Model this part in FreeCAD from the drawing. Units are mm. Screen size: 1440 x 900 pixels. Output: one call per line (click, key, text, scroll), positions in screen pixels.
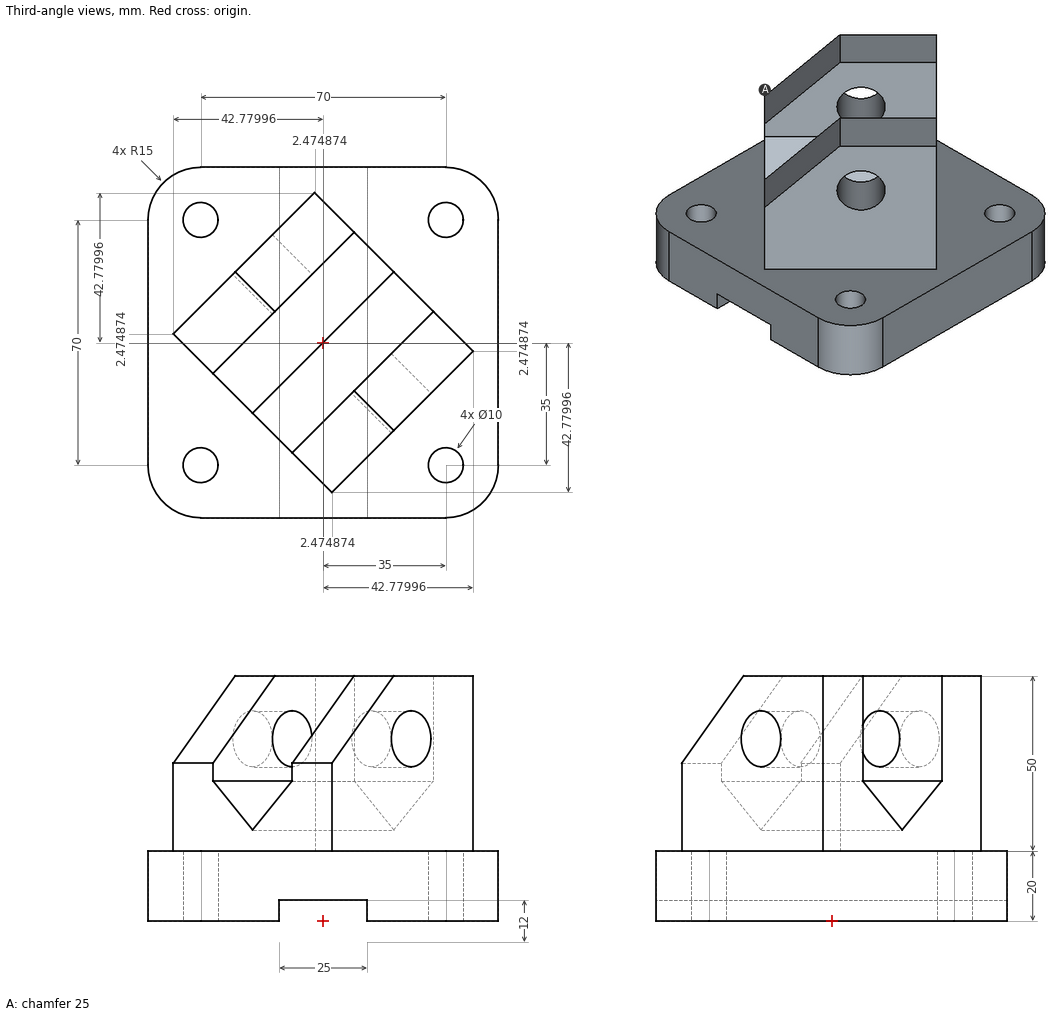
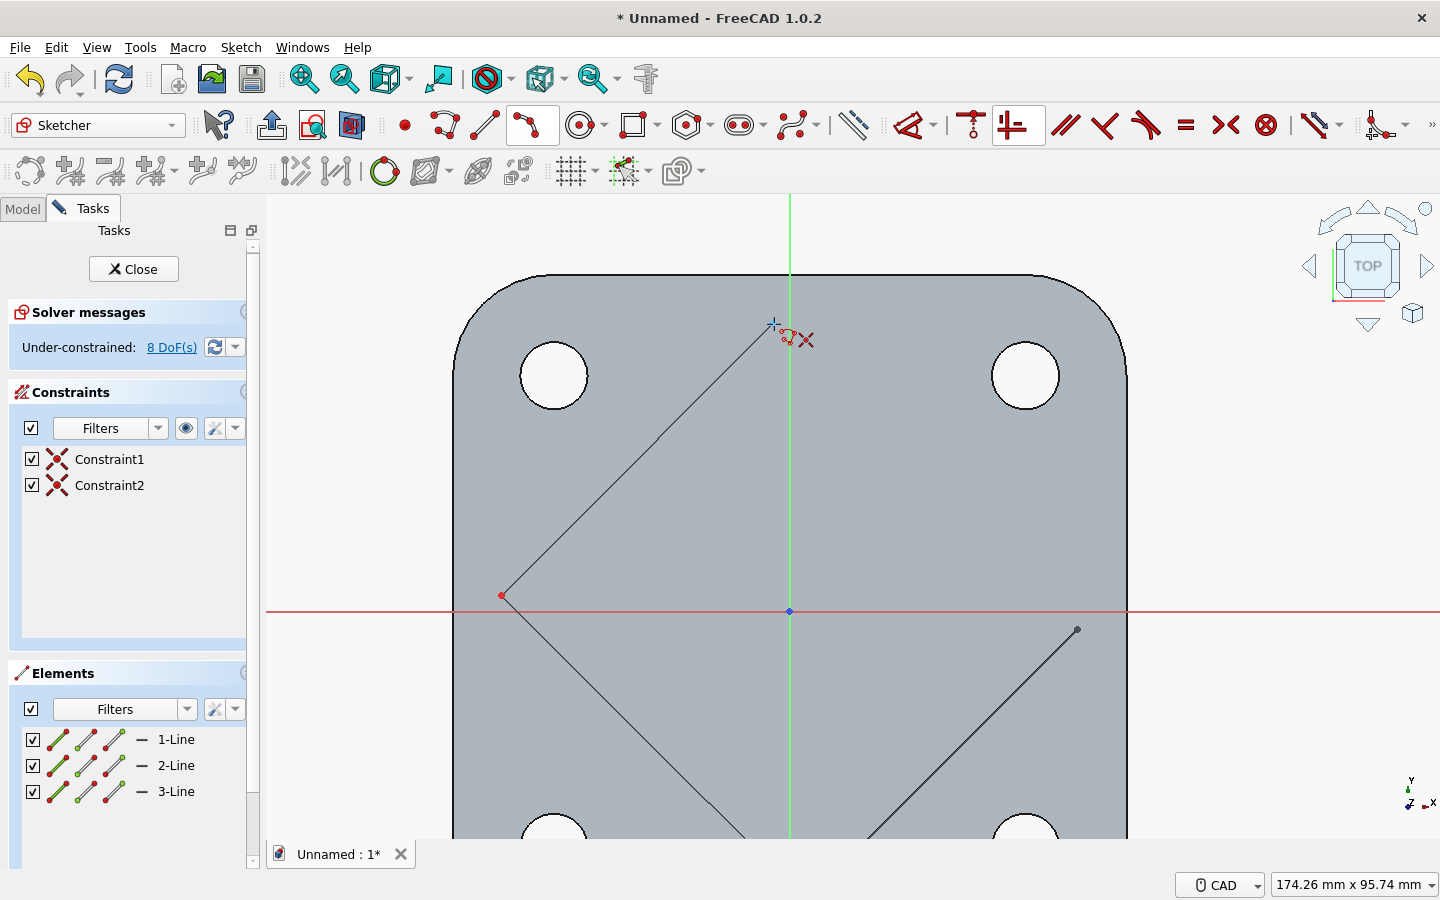
click(773, 324)
key(Escape)
key(Escape)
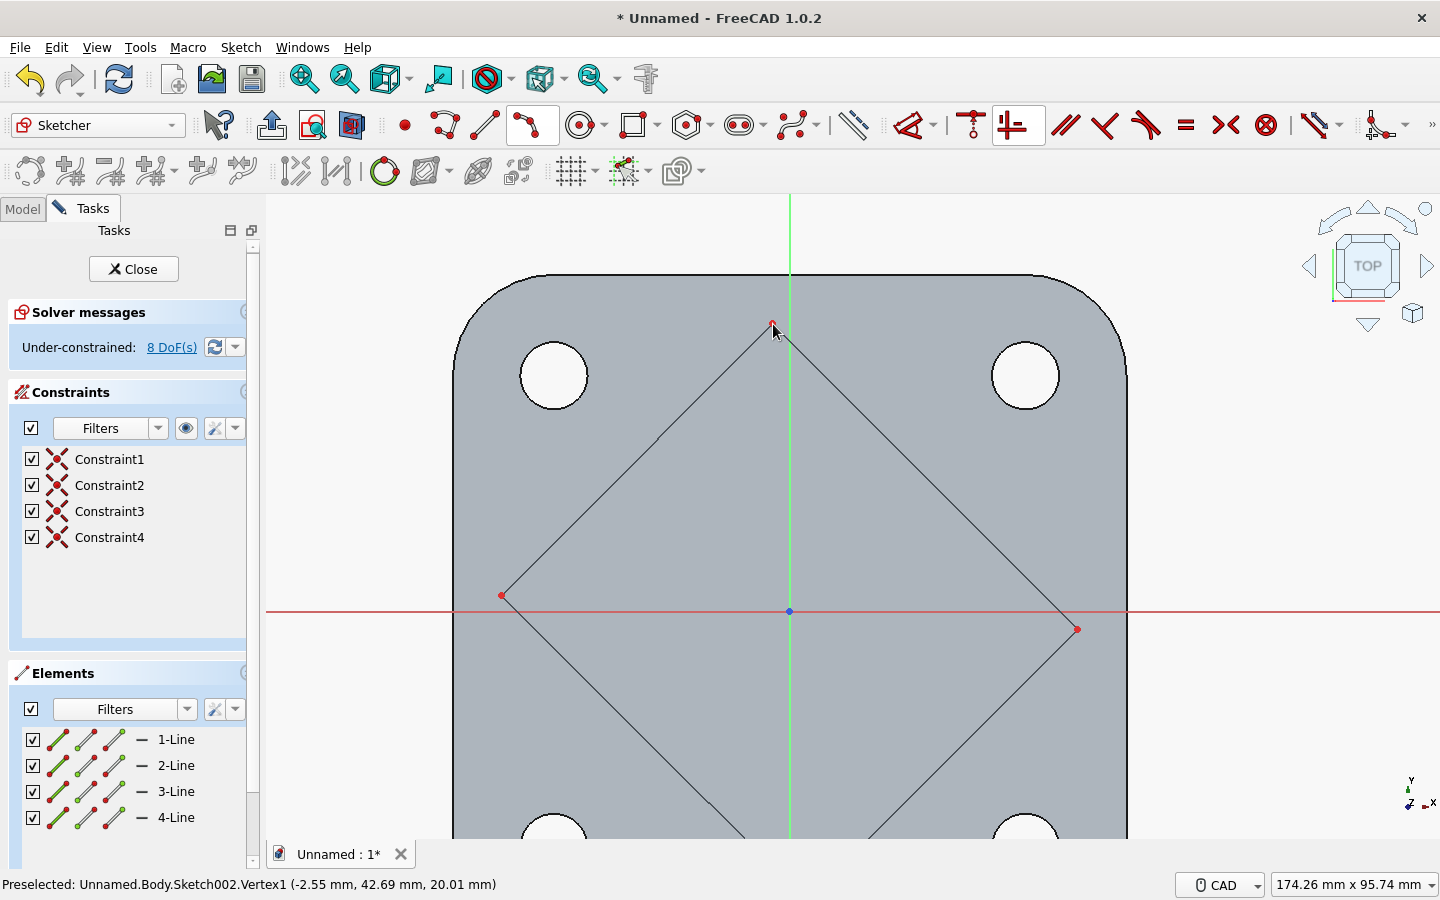
click(908, 126)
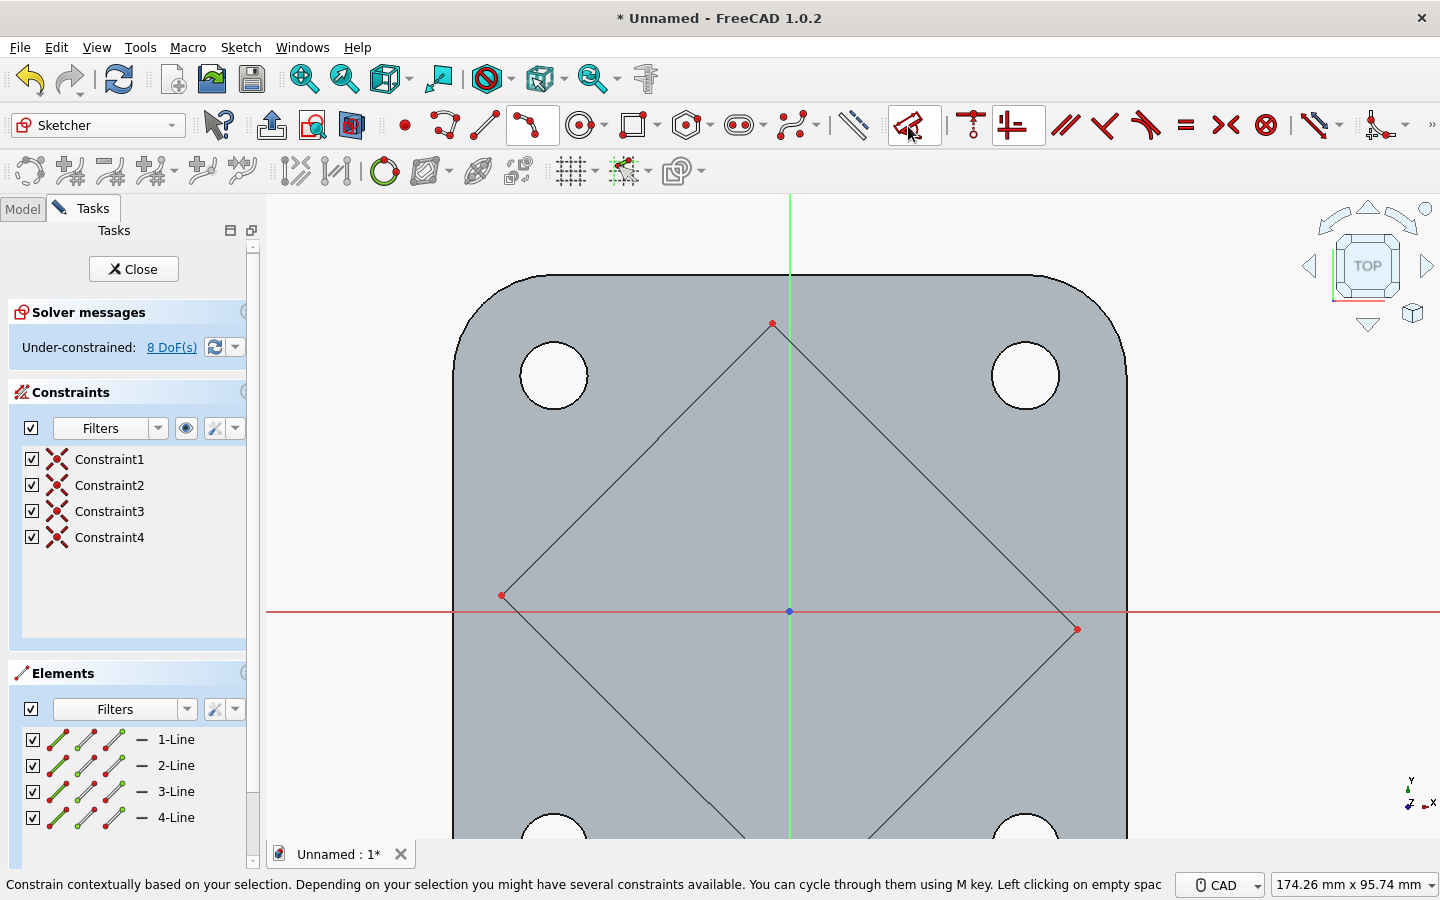
scroll(773, 324, up, 5)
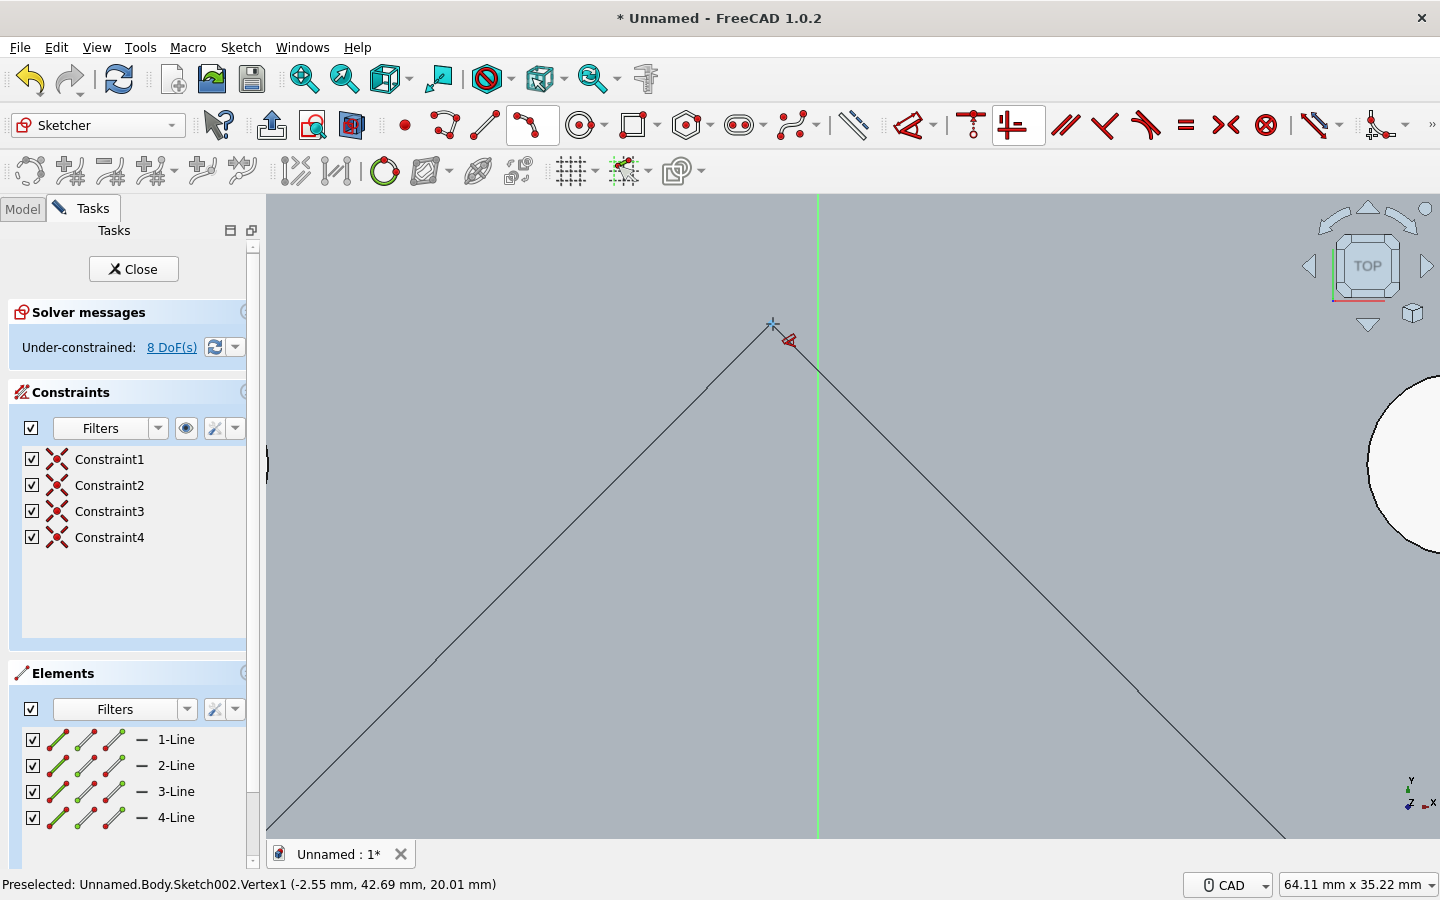
click(771, 324)
click(794, 290)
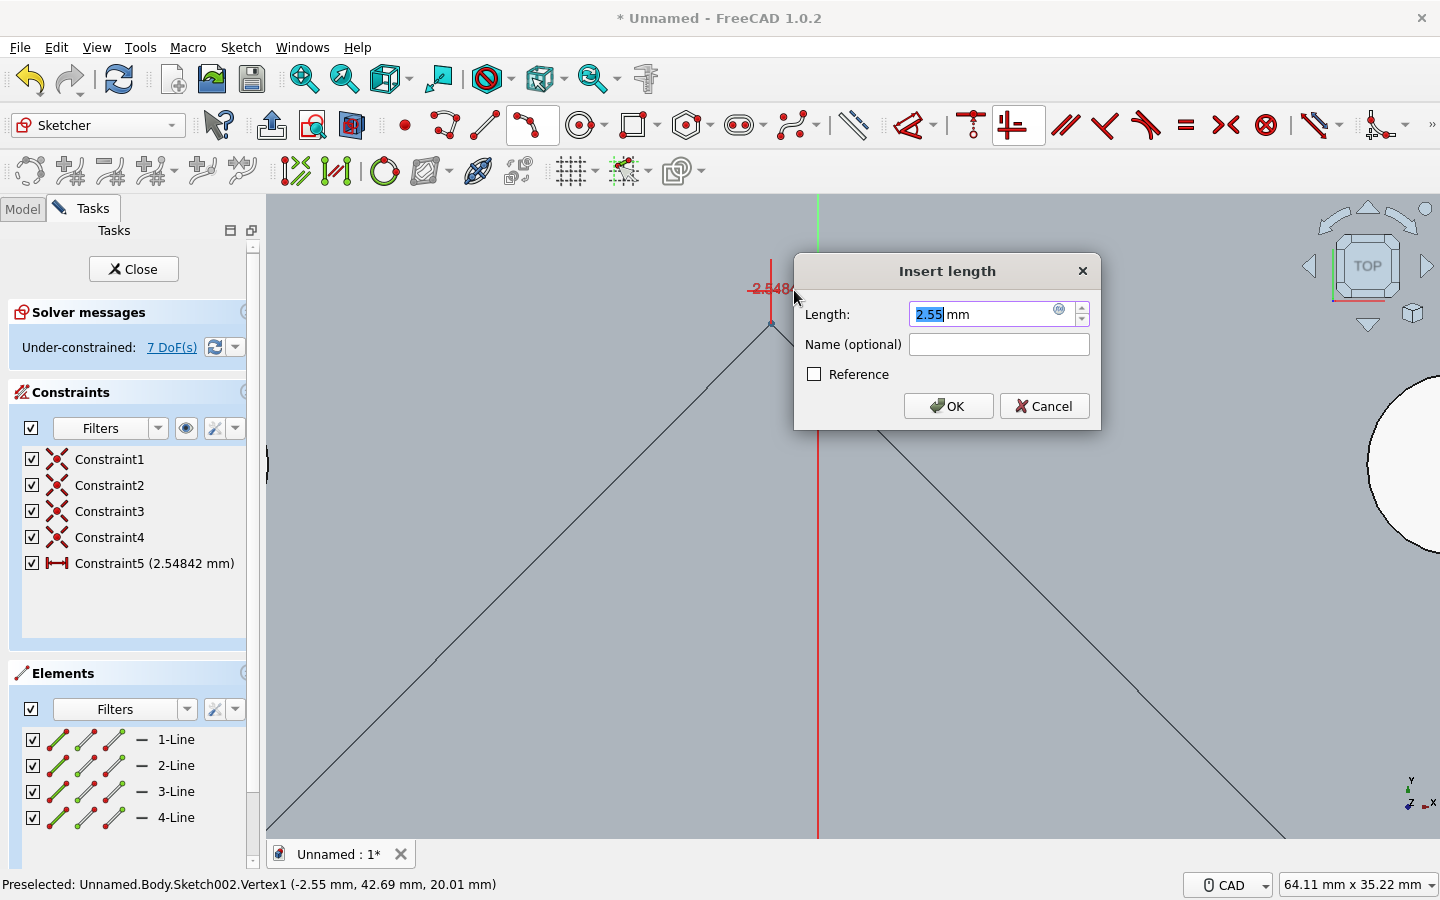
text(2.474874)
key(Return)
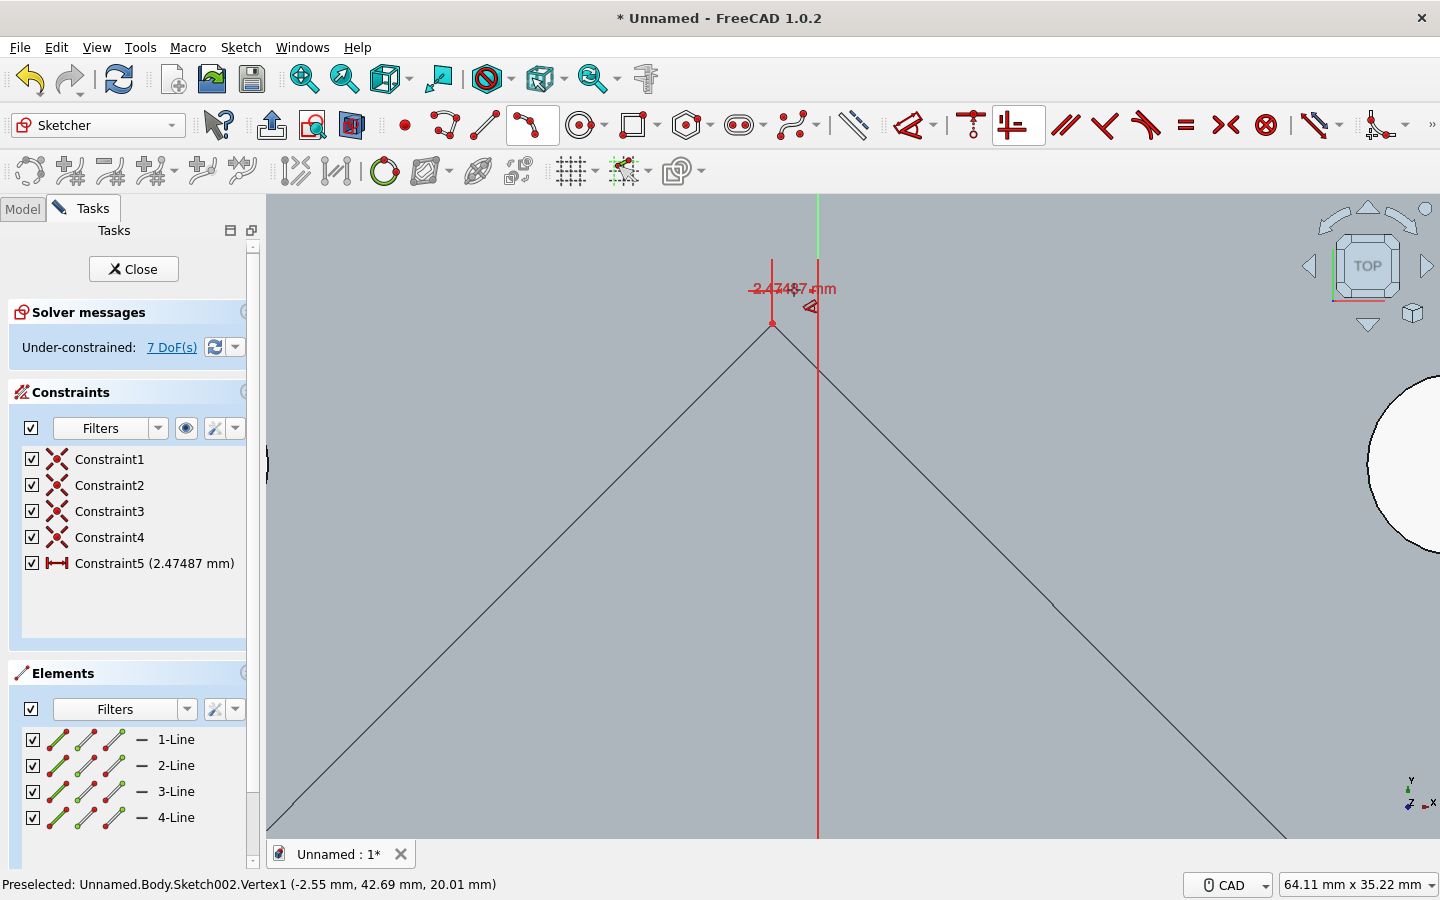
scroll(774, 324, down, 7)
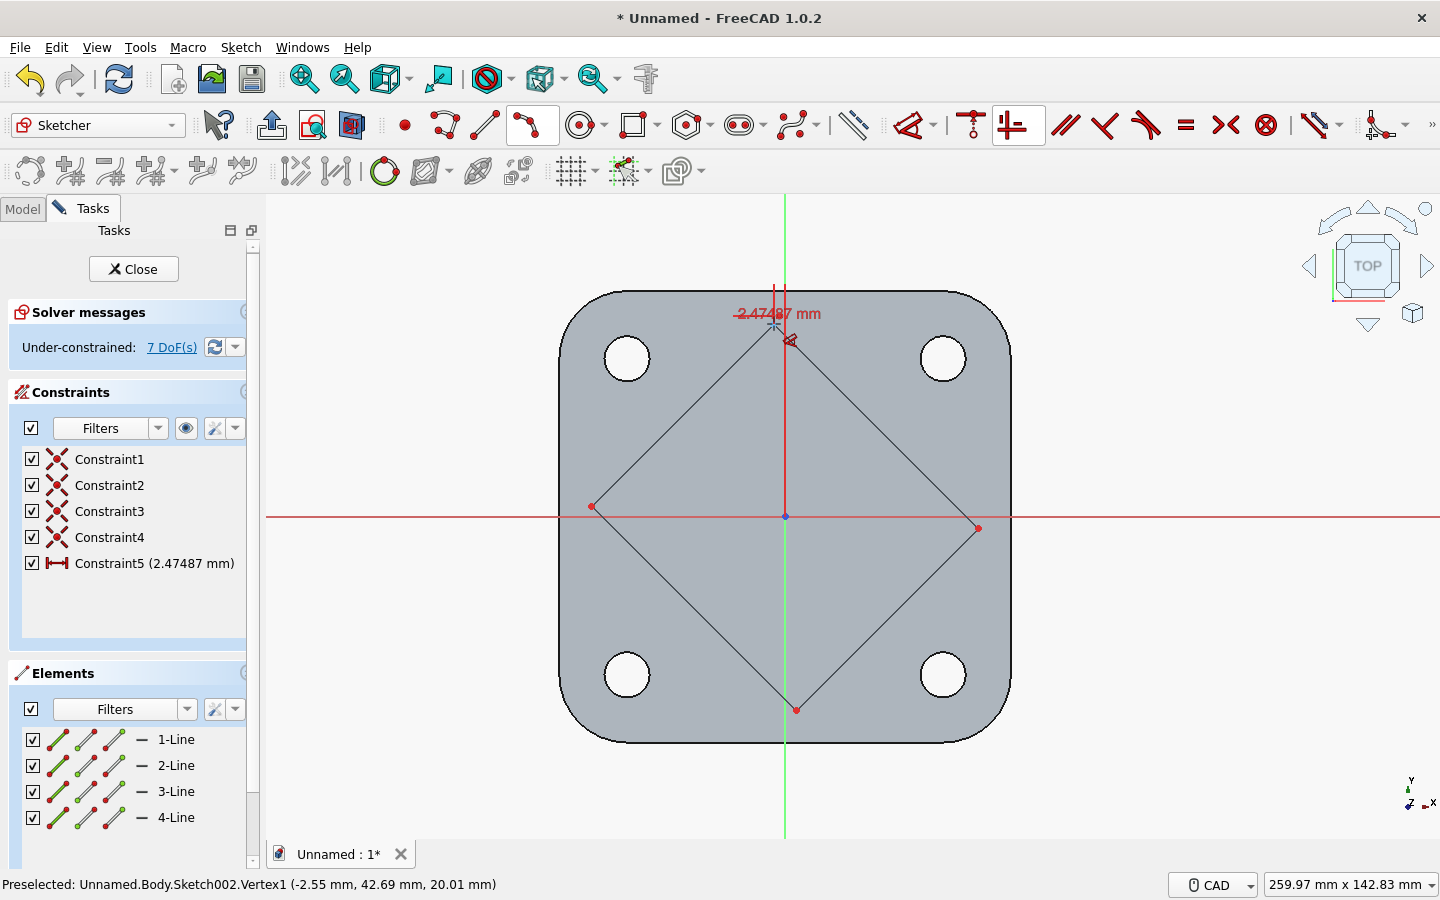
click(774, 324)
click(740, 420)